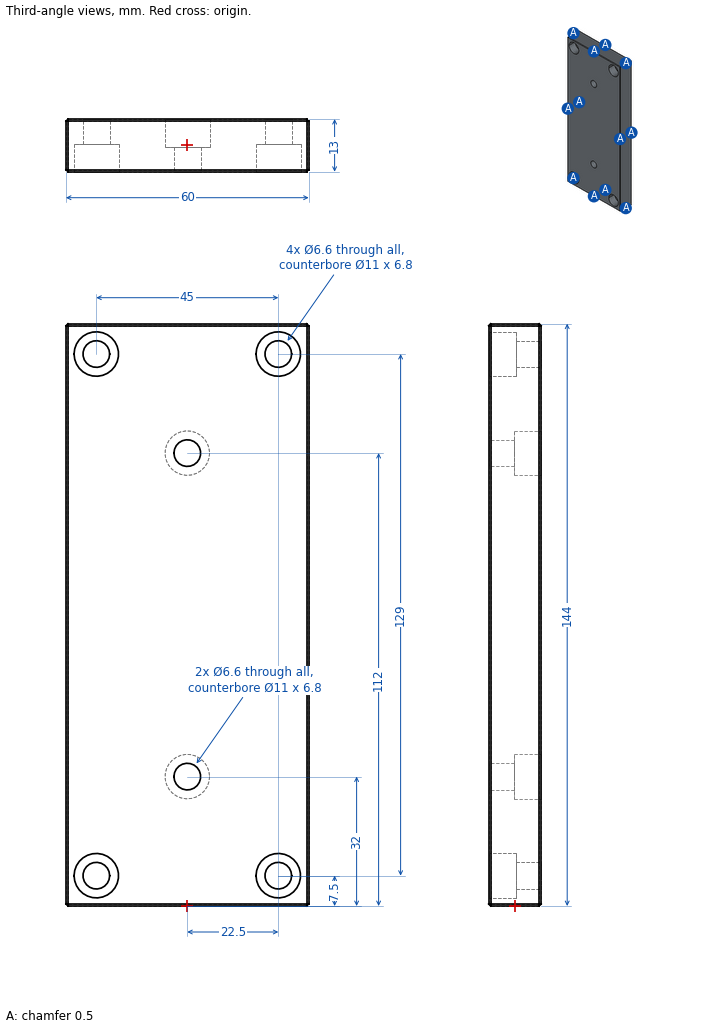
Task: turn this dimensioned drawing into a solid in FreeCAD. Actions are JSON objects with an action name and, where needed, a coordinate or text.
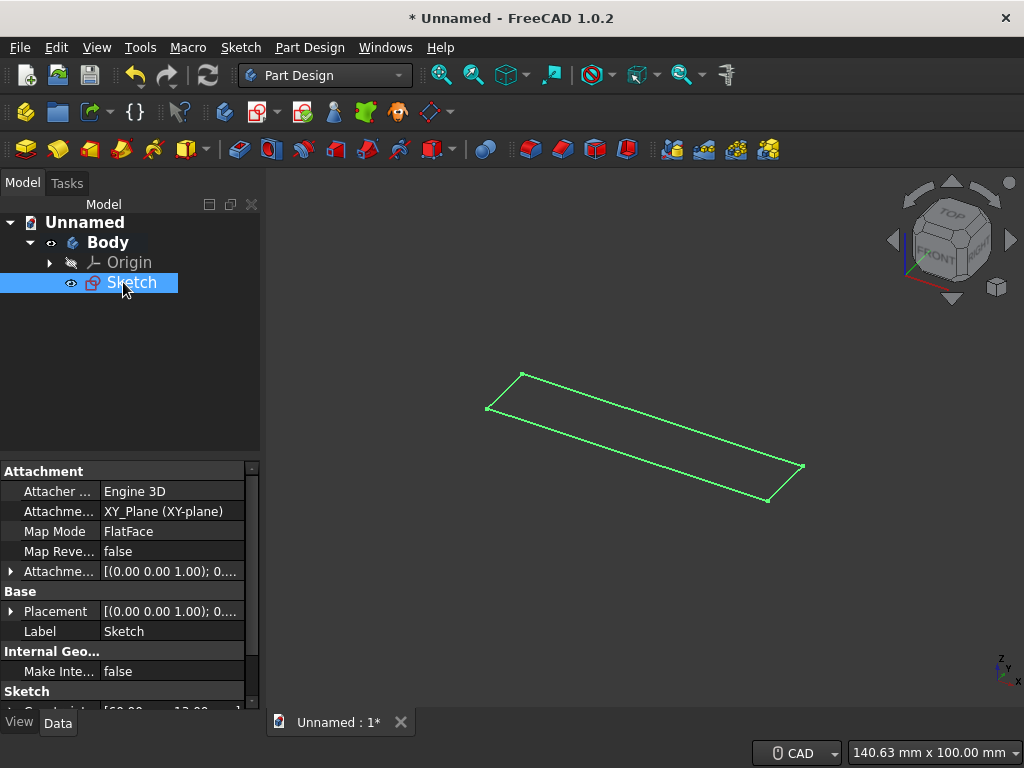
{"action": "left_click", "coordinate": [26, 150]}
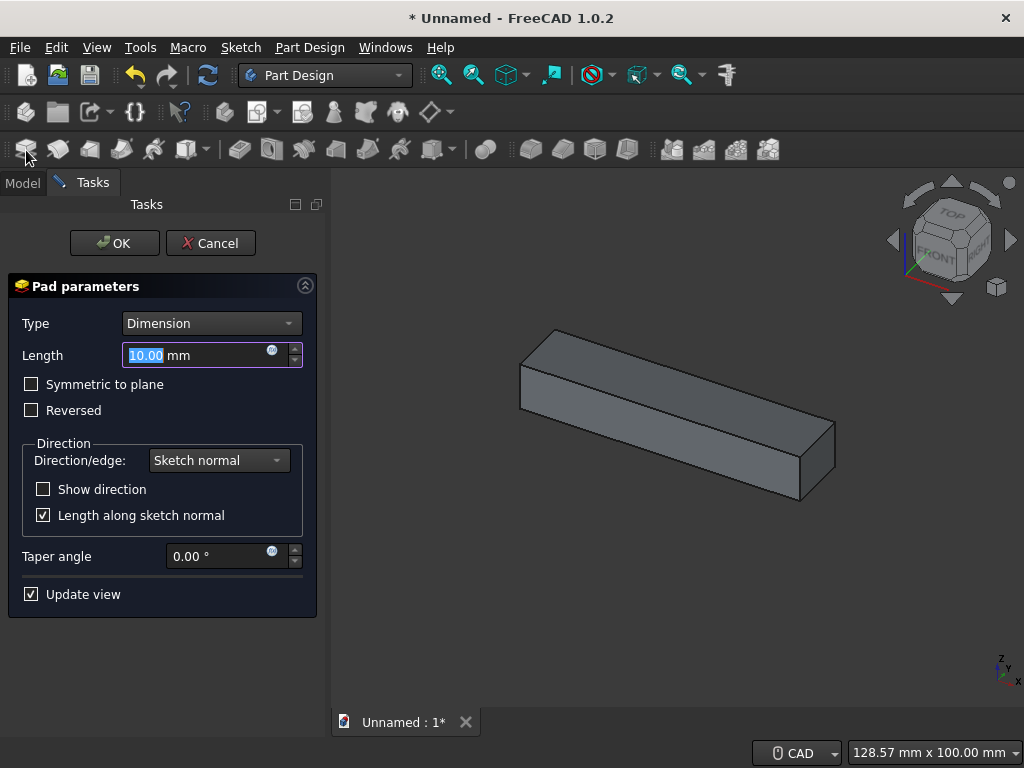
{"action": "type", "text": "144"}
{"action": "key", "text": "Tab"}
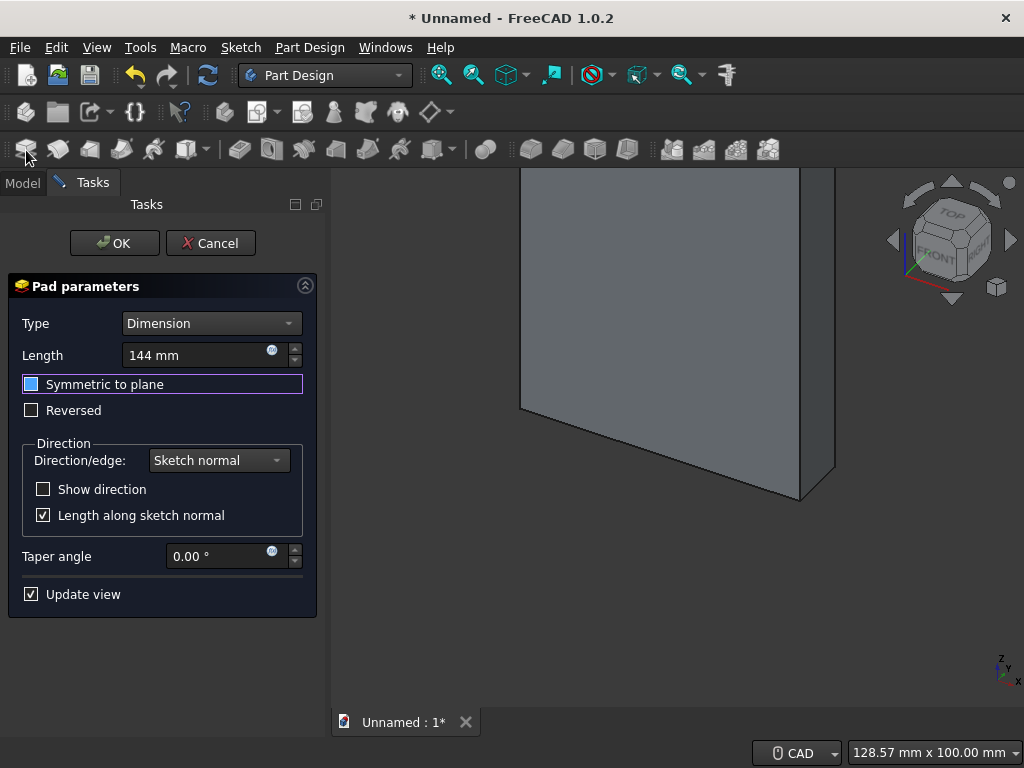
{"action": "left_click", "coordinate": [115, 243]}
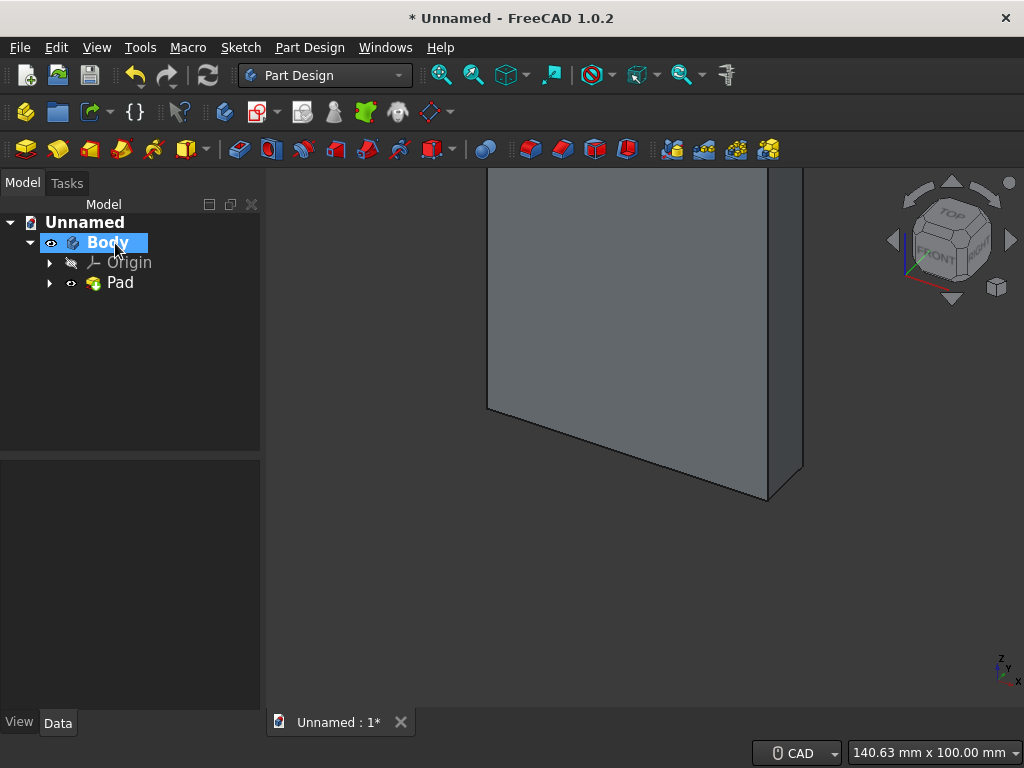
{"action": "key", "text": "v f"}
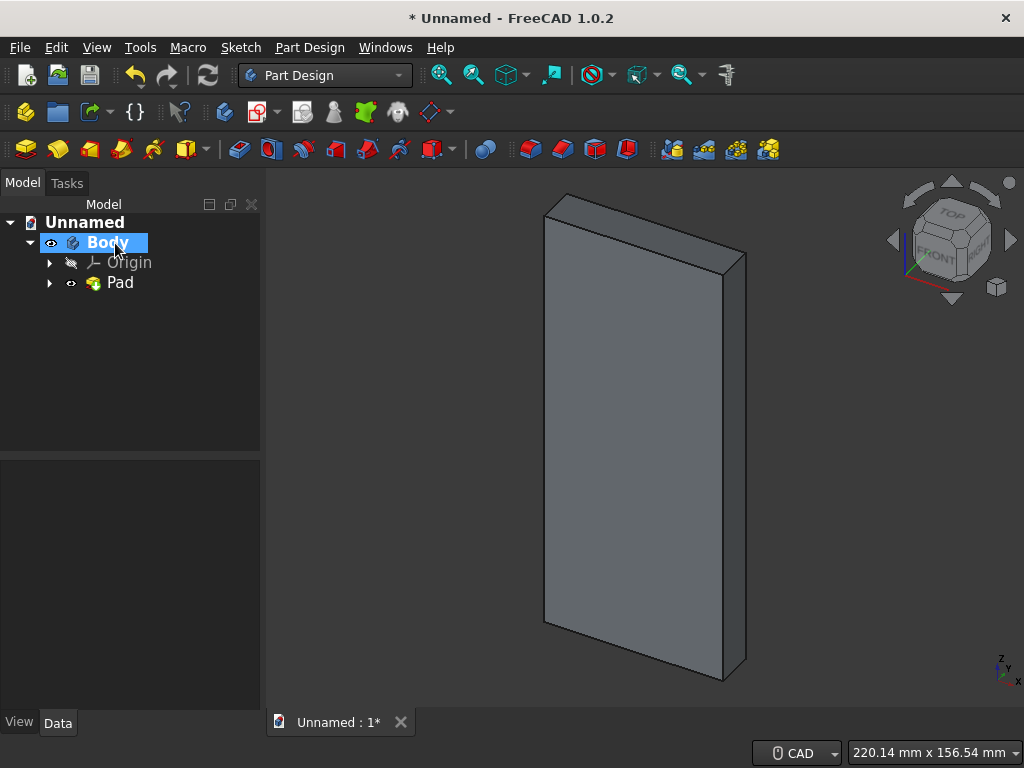
{"action": "key", "text": "4"}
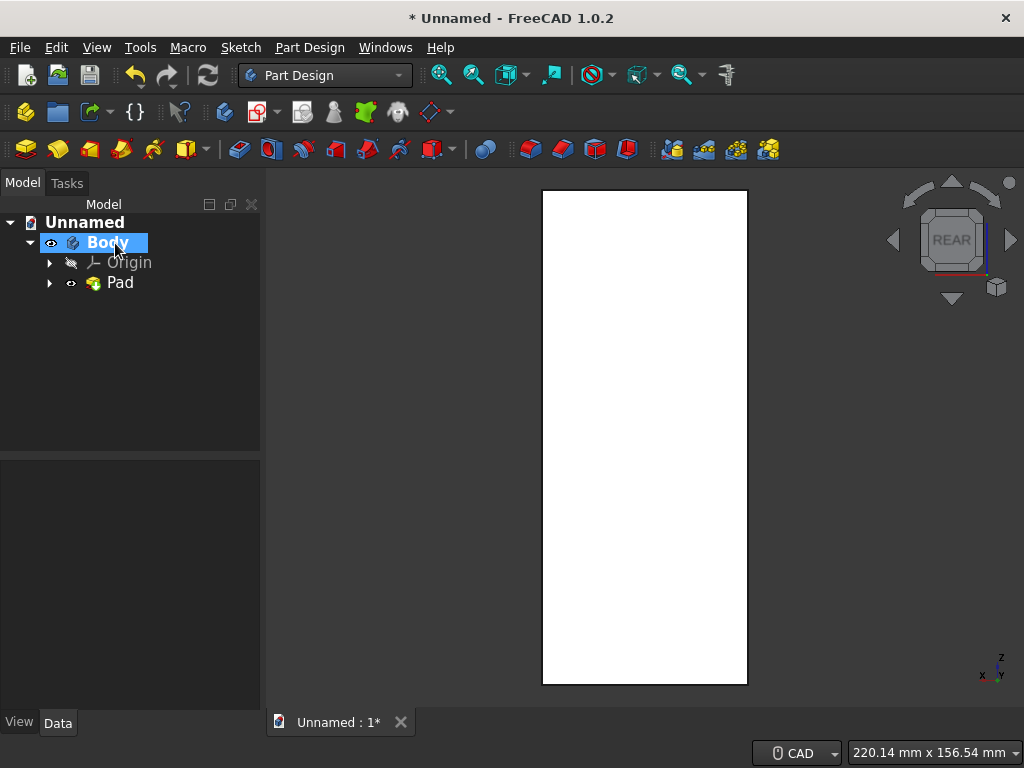
{"action": "left_click", "coordinate": [645, 295]}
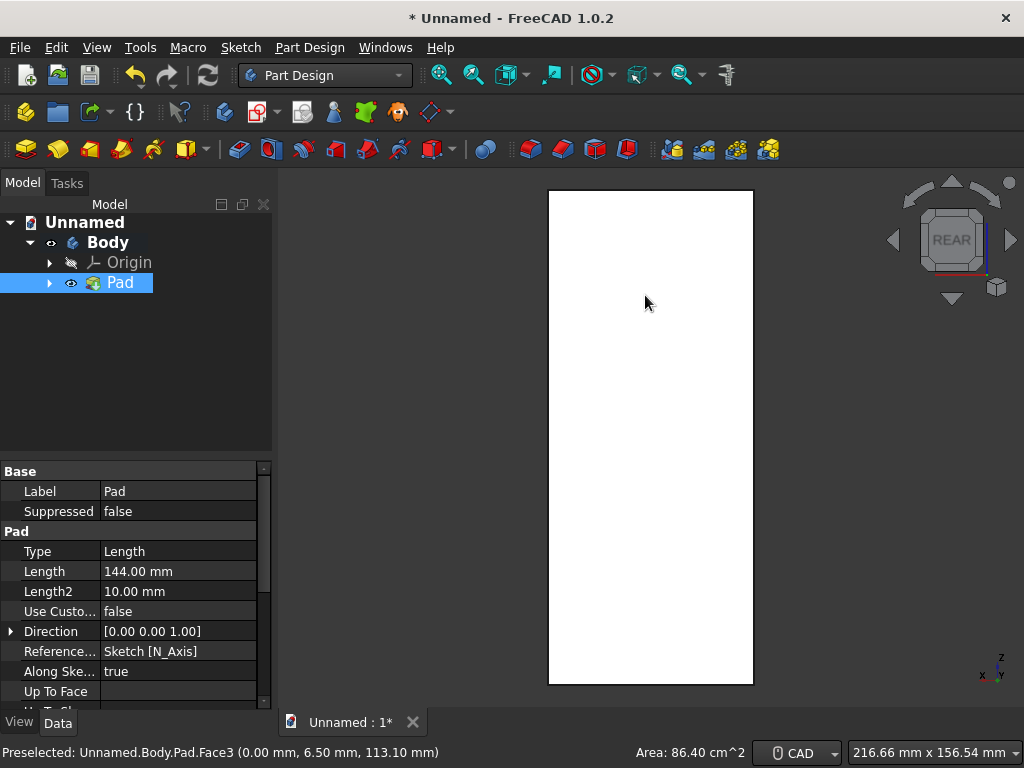
{"action": "left_click", "coordinate": [258, 112]}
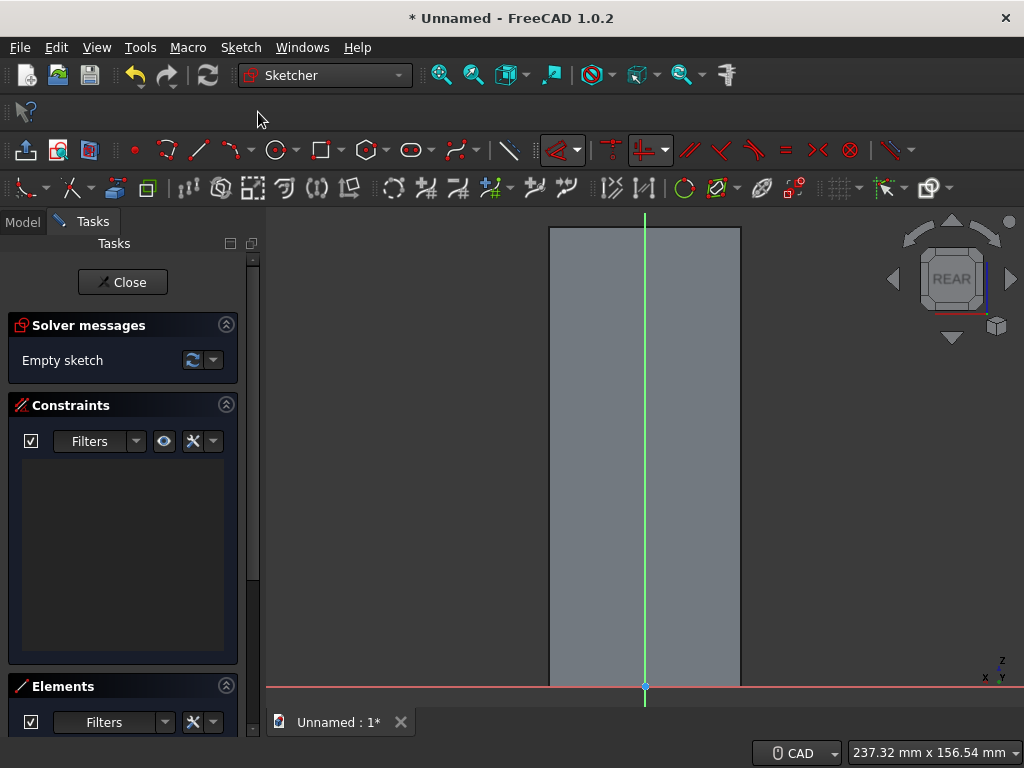
{"action": "scroll", "coordinate": [294, 250], "scroll_direction": "down", "scroll_amount": 1}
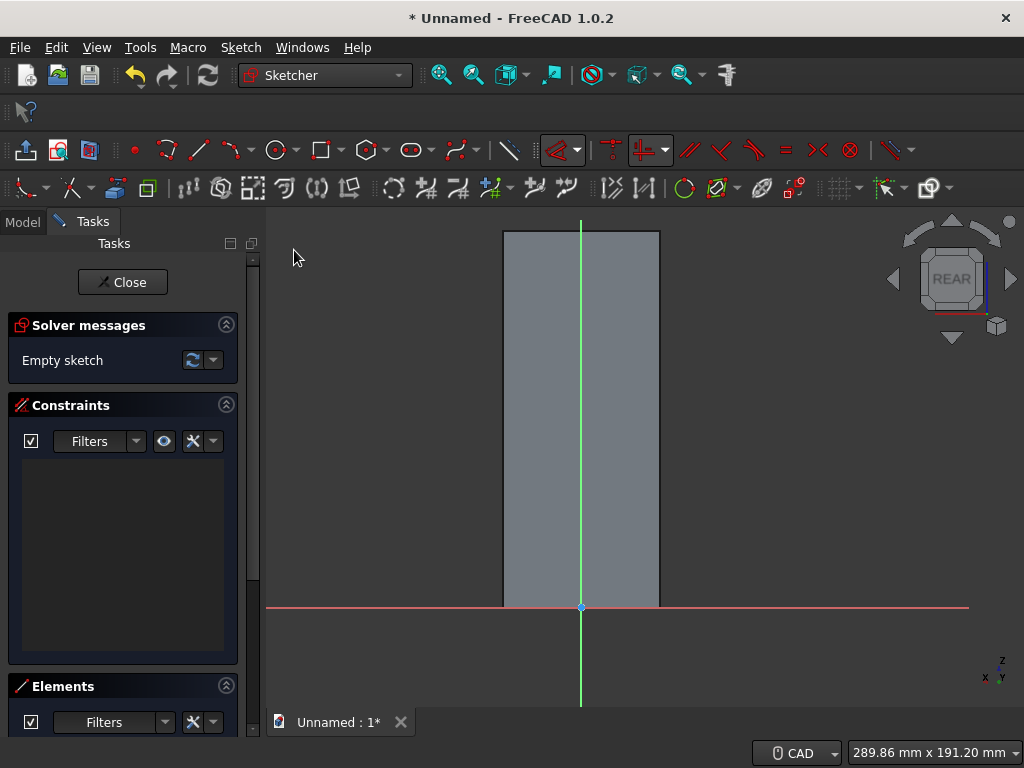
{"action": "key", "text": "g c"}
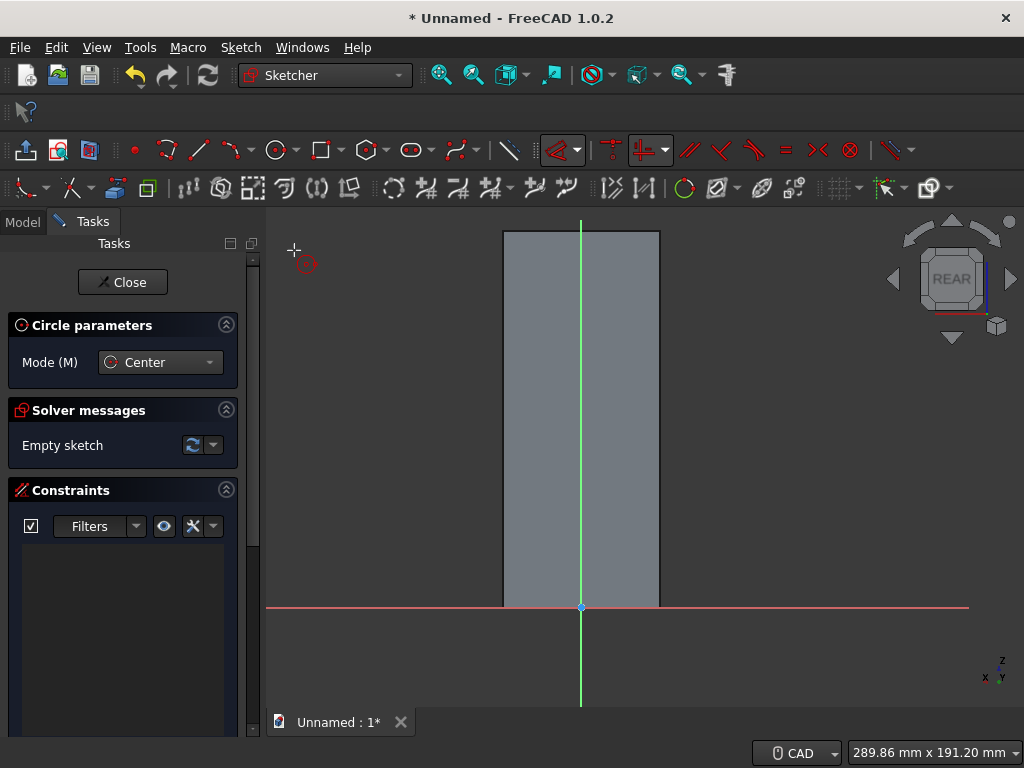
{"action": "scroll", "coordinate": [581, 524], "scroll_direction": "up", "scroll_amount": 5}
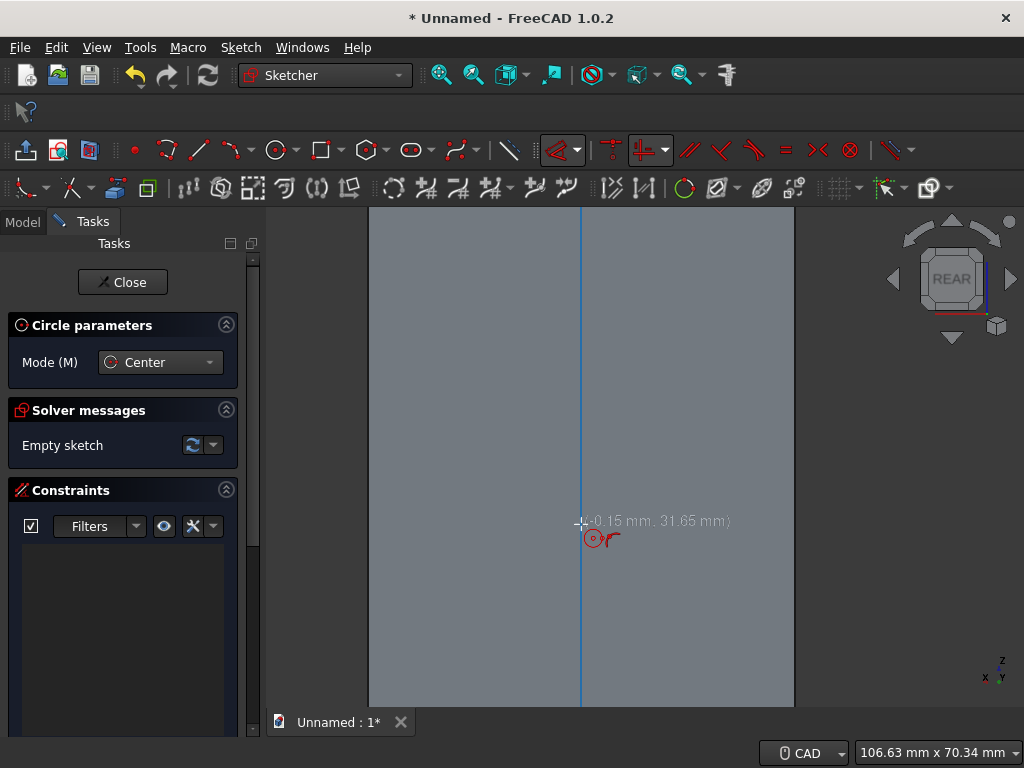
{"action": "left_click", "coordinate": [581, 523]}
{"action": "left_click", "coordinate": [598, 507]}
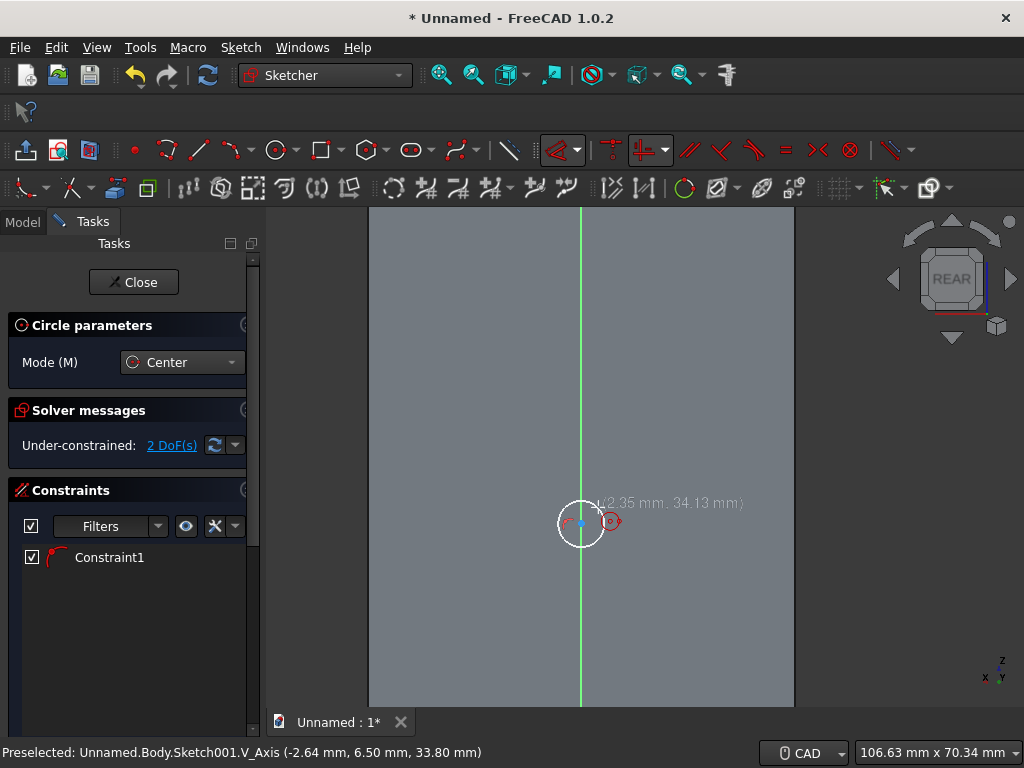
{"action": "scroll", "coordinate": [574, 525], "scroll_direction": "down", "scroll_amount": 5}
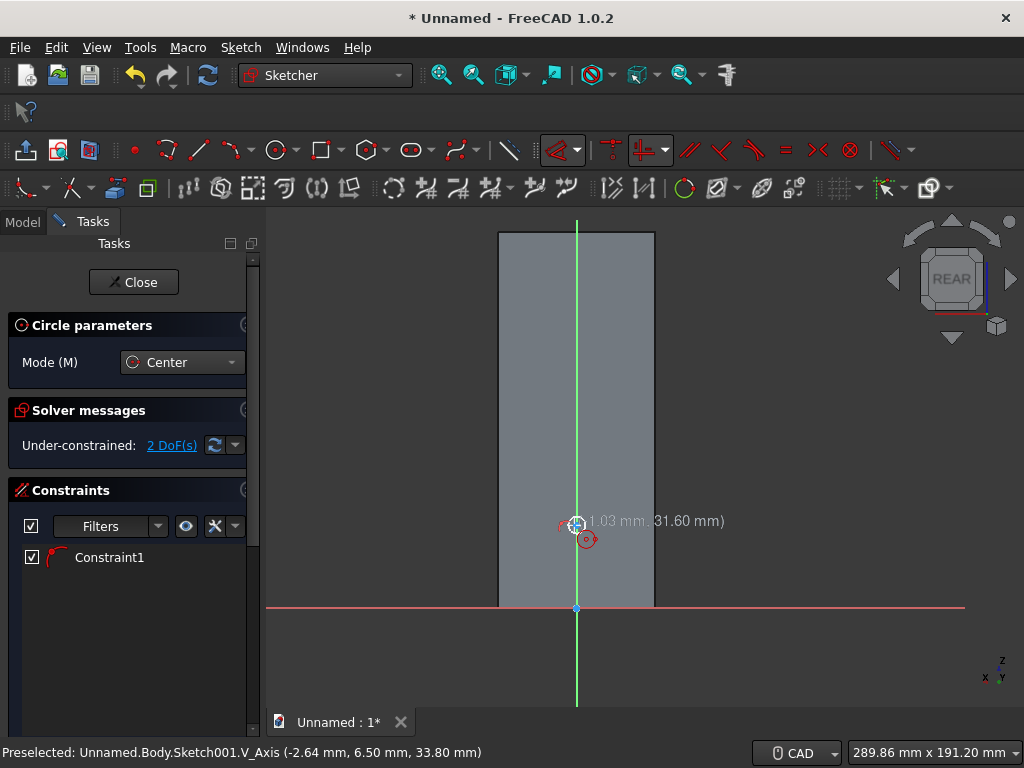
{"action": "scroll", "coordinate": [577, 316], "scroll_direction": "up", "scroll_amount": 5}